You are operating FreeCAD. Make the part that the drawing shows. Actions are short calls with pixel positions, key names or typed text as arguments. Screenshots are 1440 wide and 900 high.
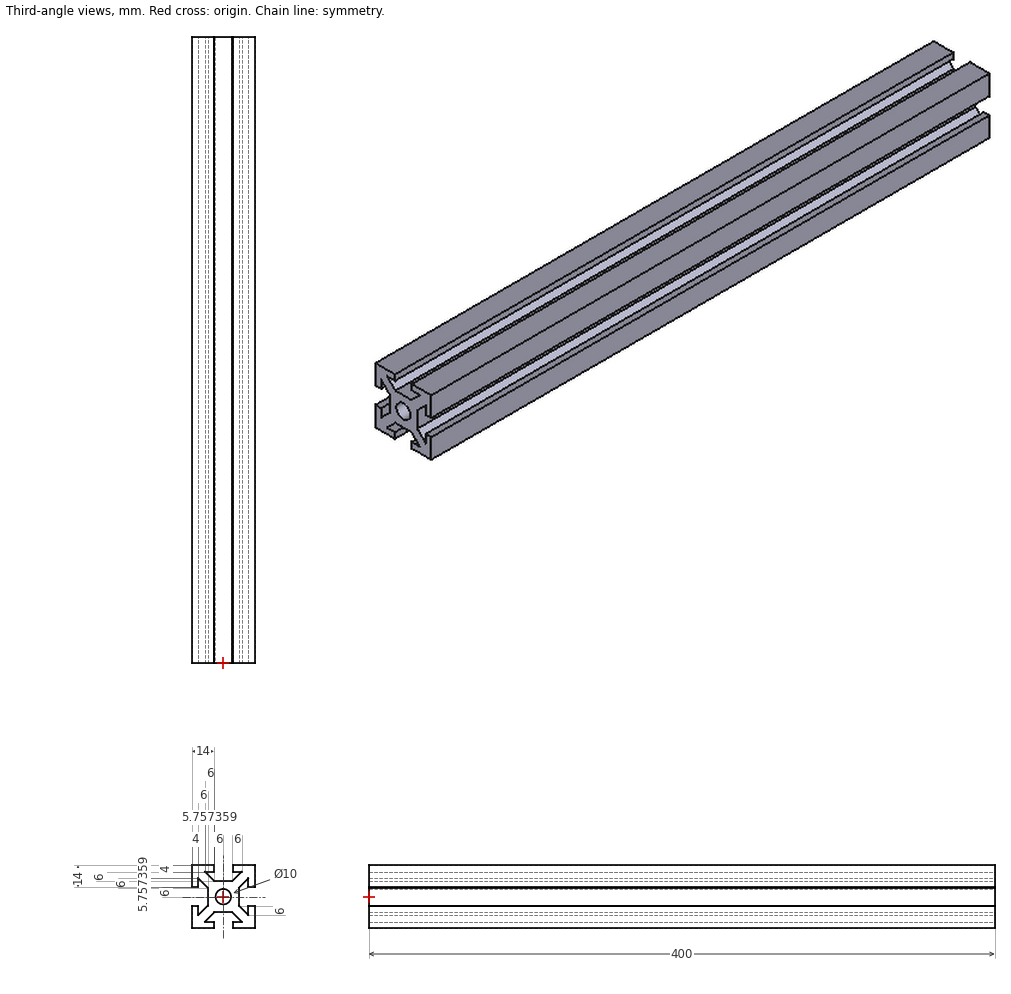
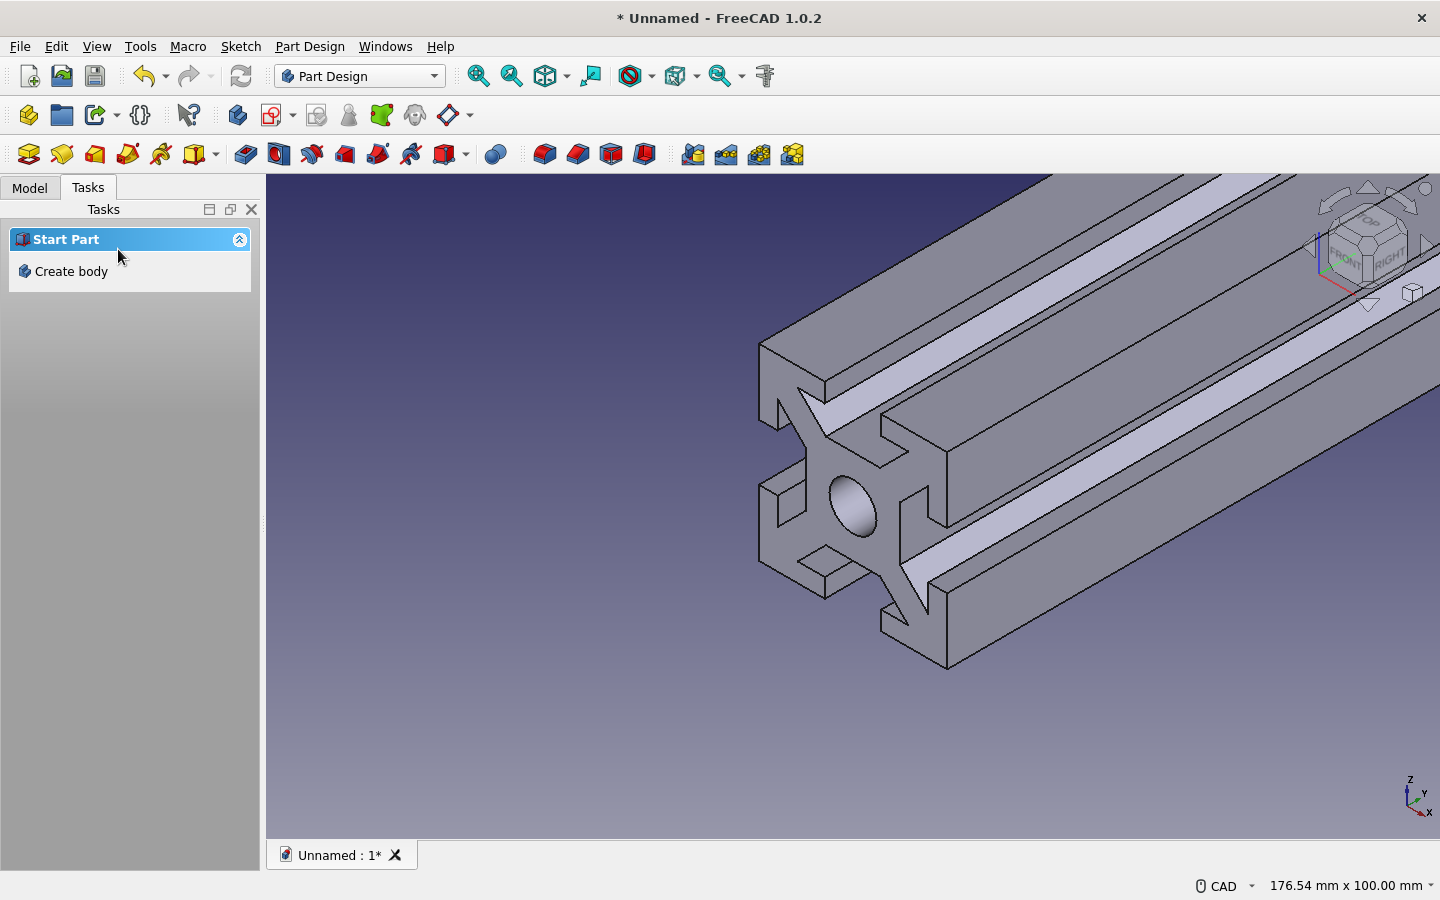
key(v)
key(f)